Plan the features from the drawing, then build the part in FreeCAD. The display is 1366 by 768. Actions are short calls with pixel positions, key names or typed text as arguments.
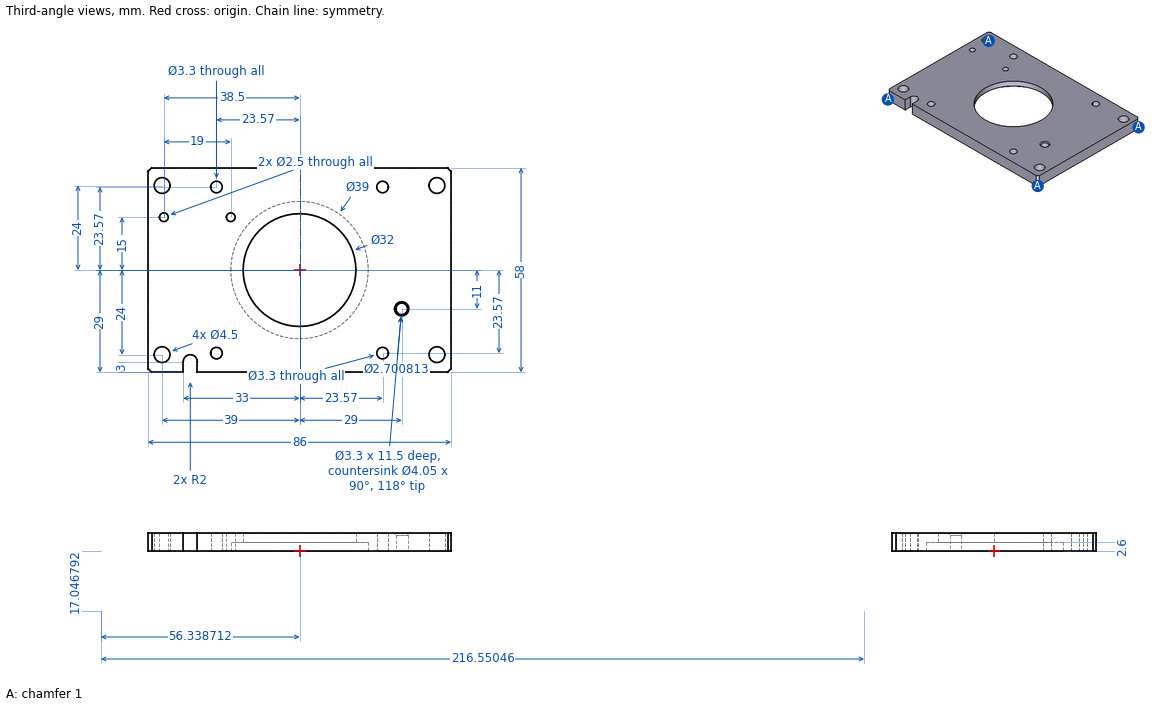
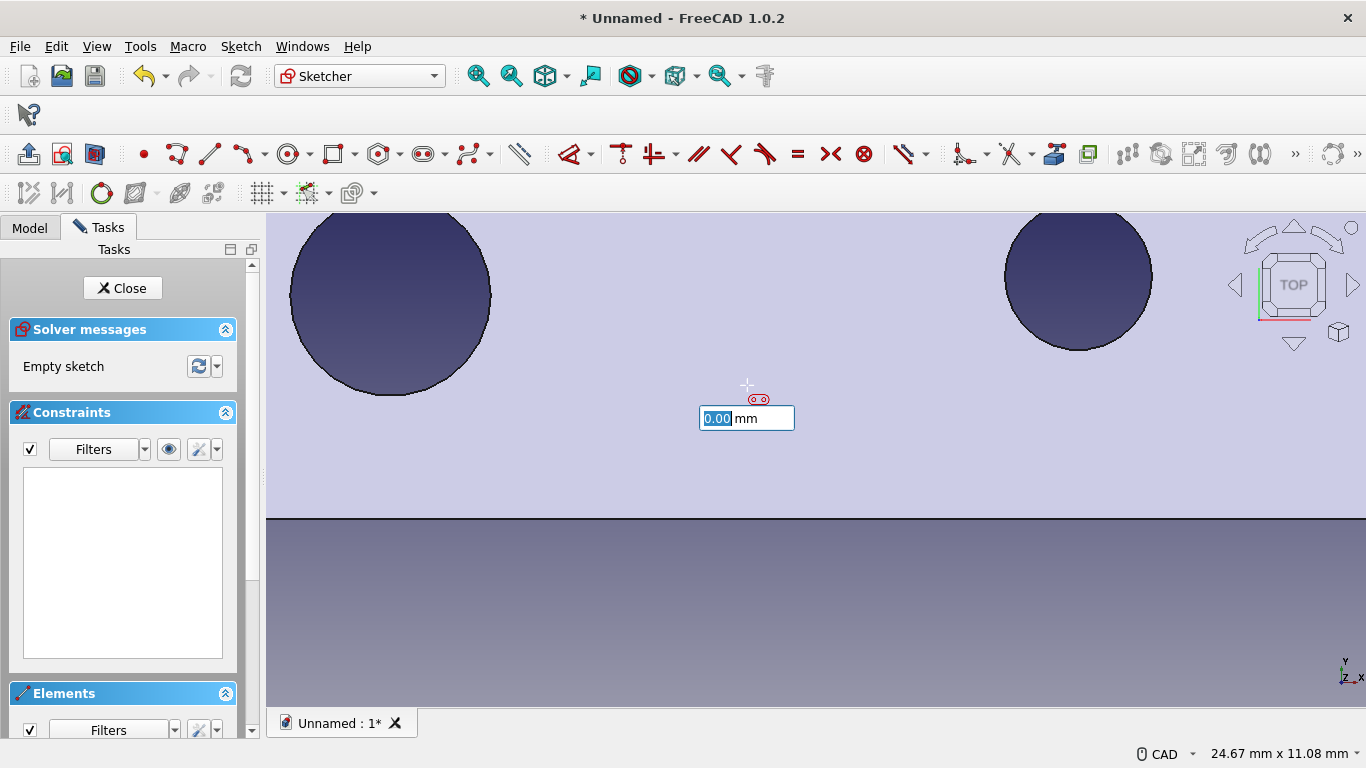
click(658, 452)
key(Escape)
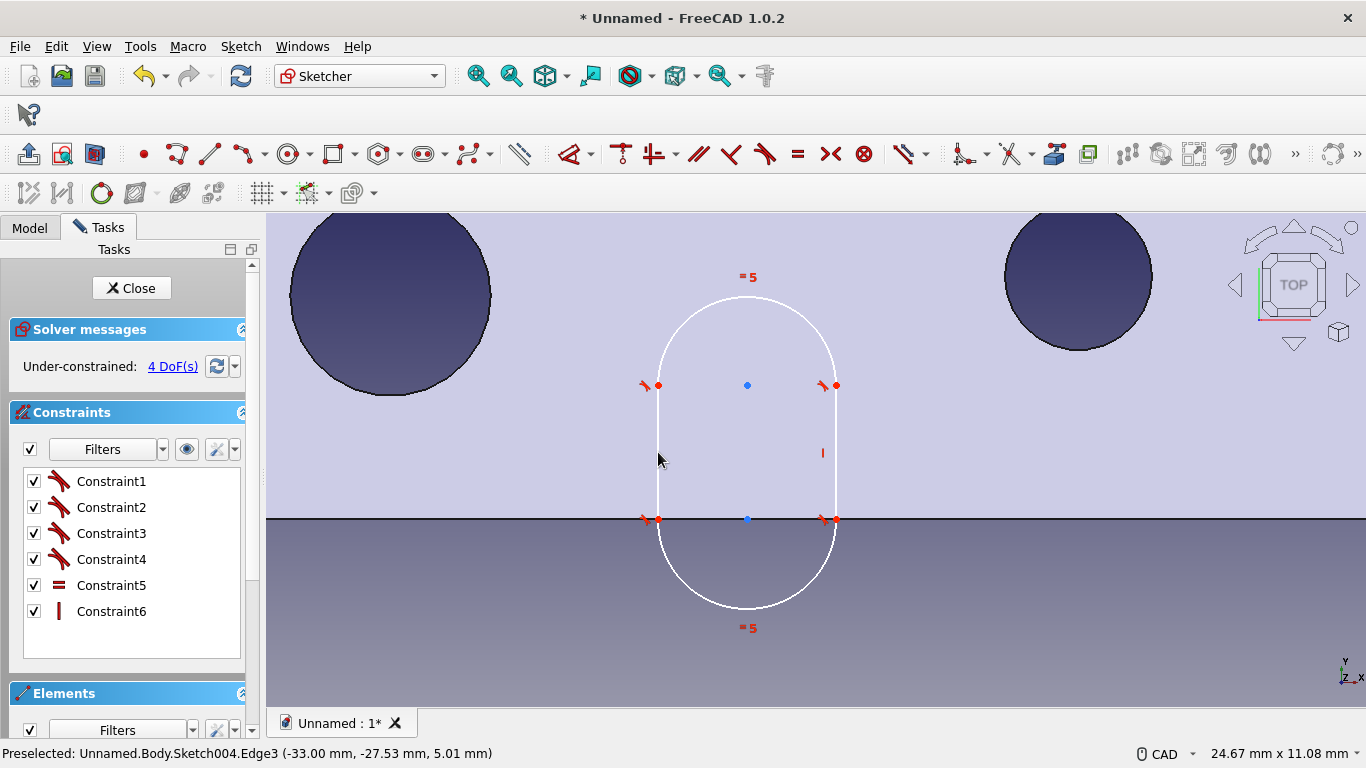
key(d)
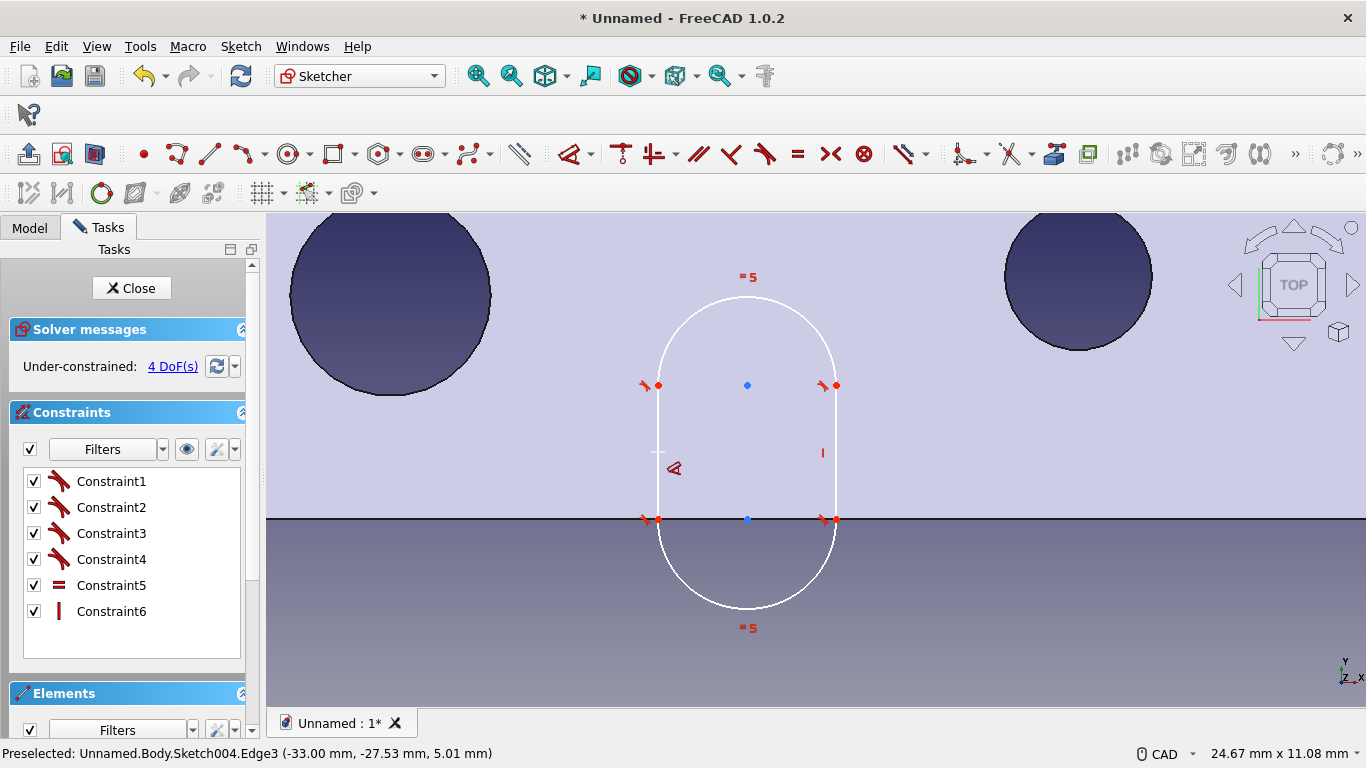
click(695, 592)
click(676, 618)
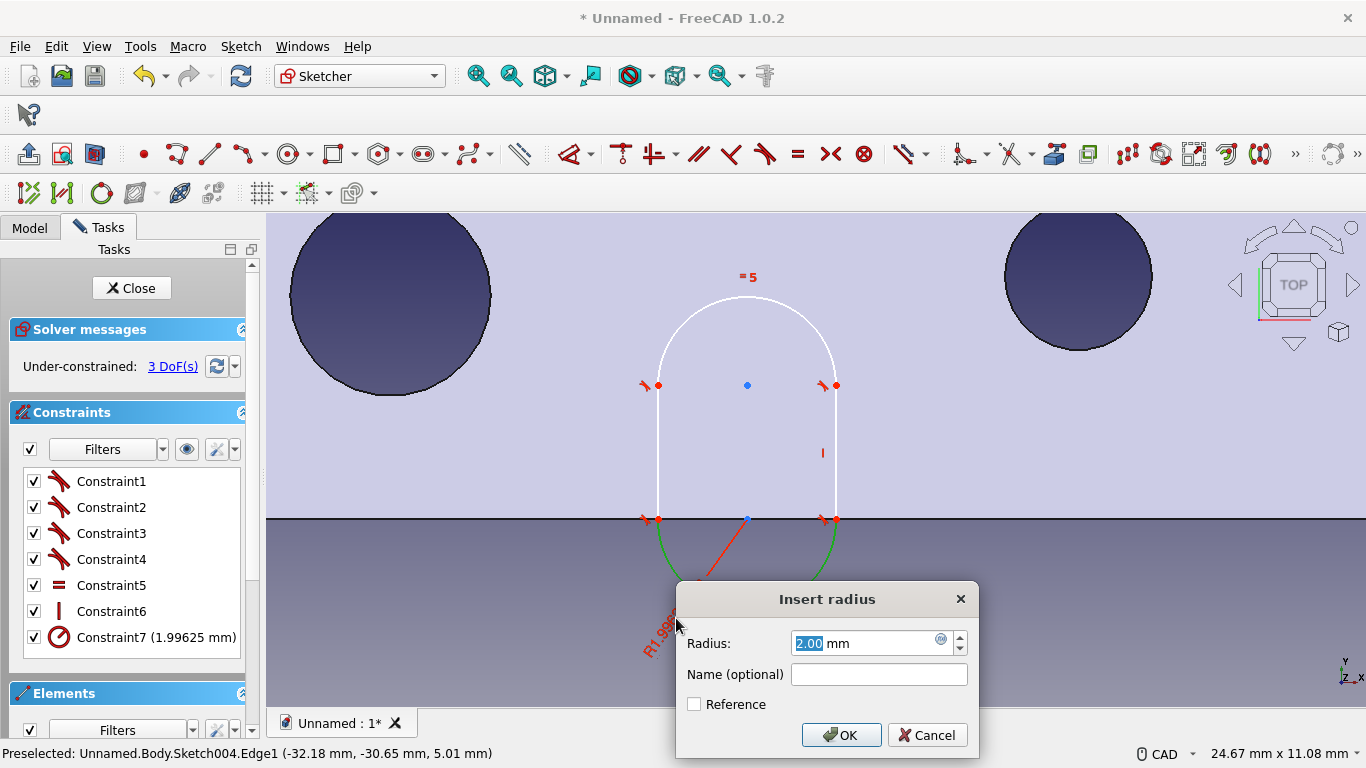
text(2)
key(Return)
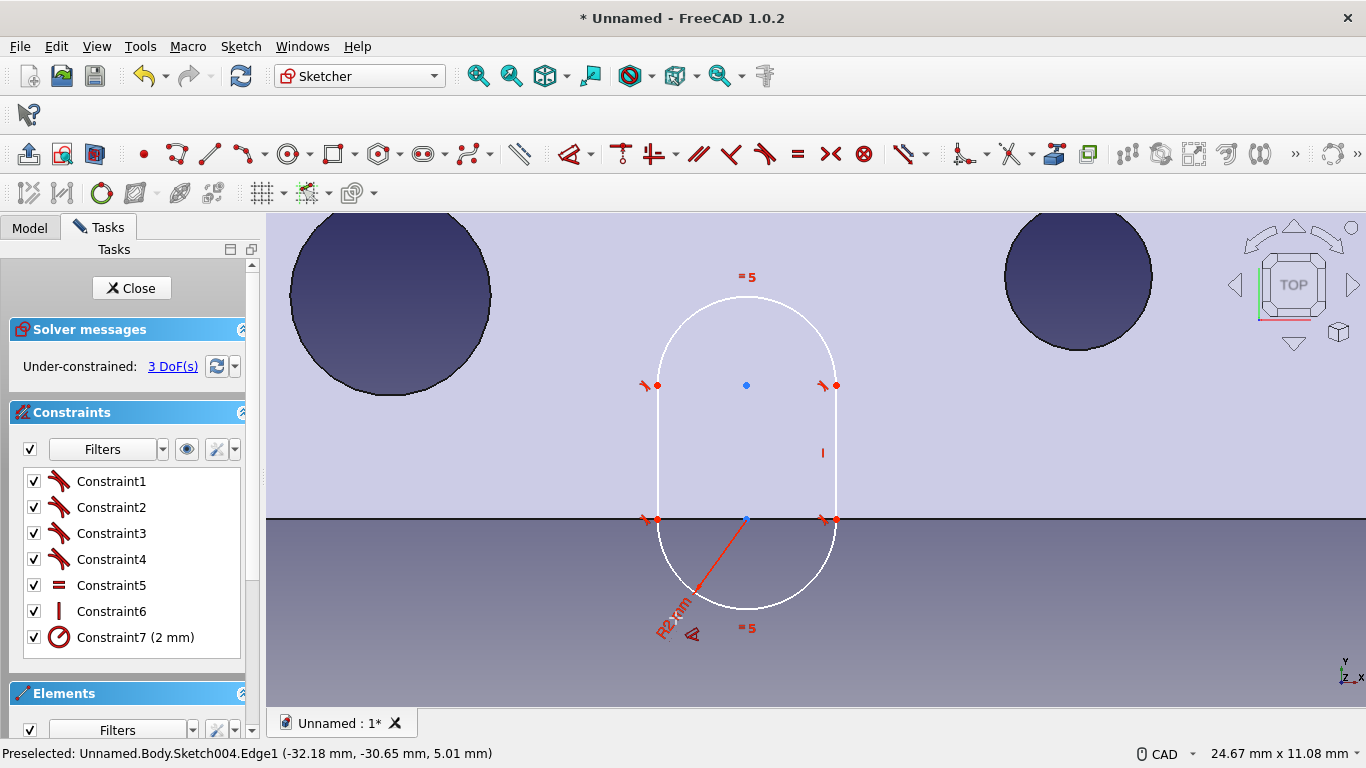
click(658, 480)
click(624, 453)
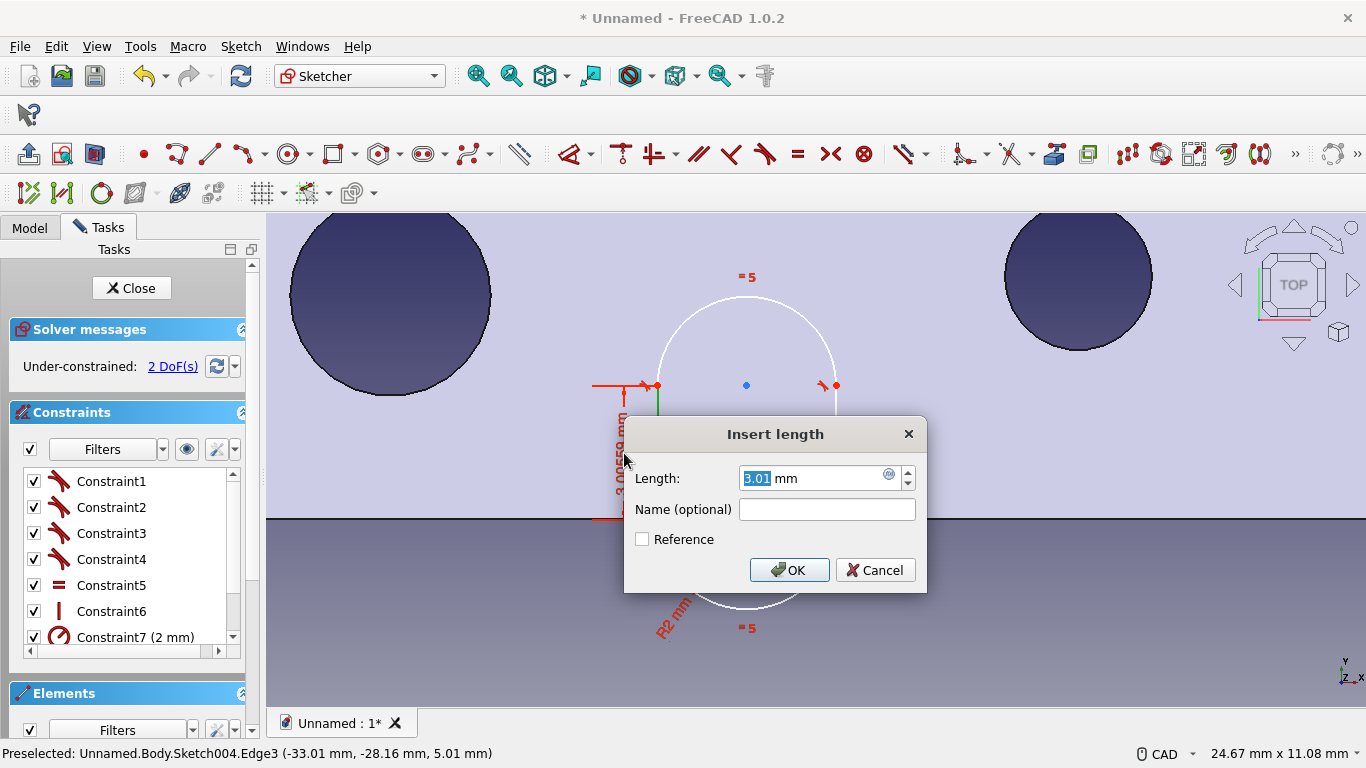
text(3)
key(Return)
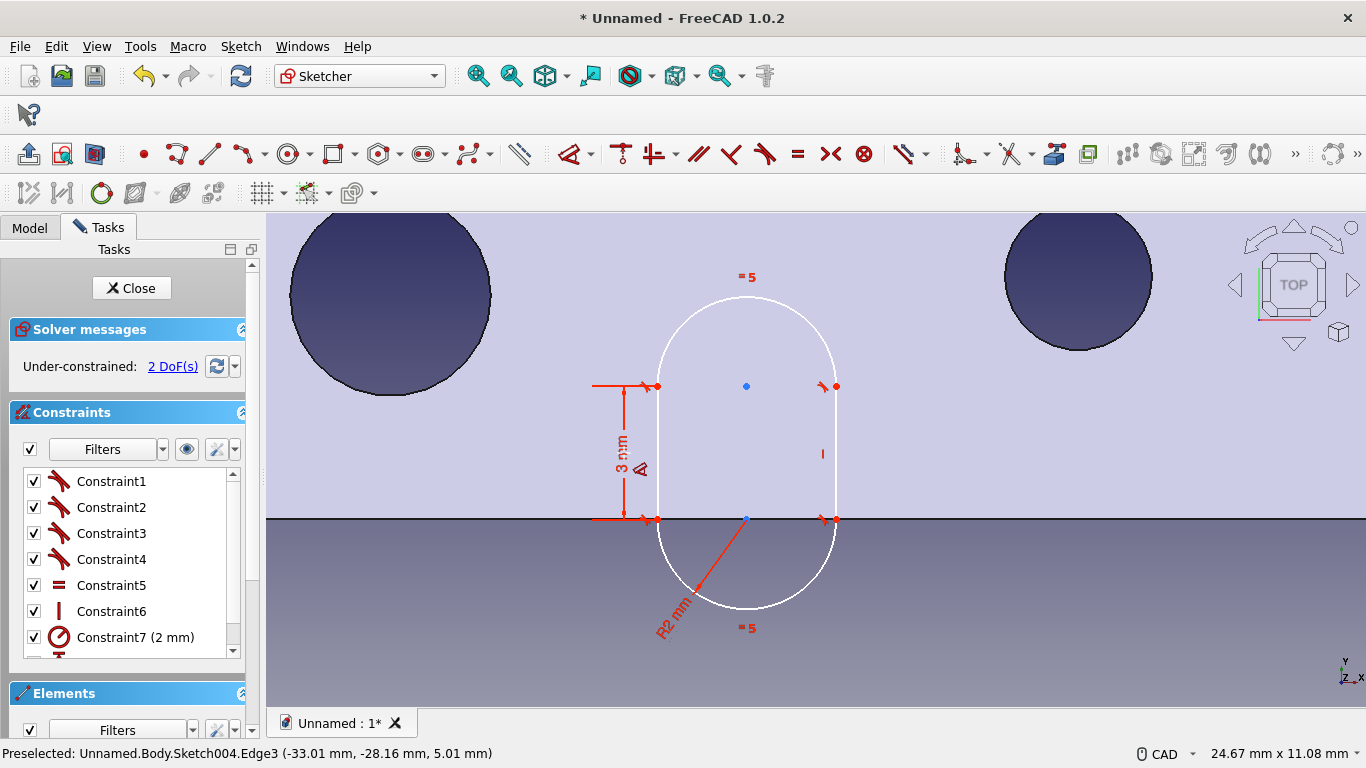
click(658, 520)
click(929, 554)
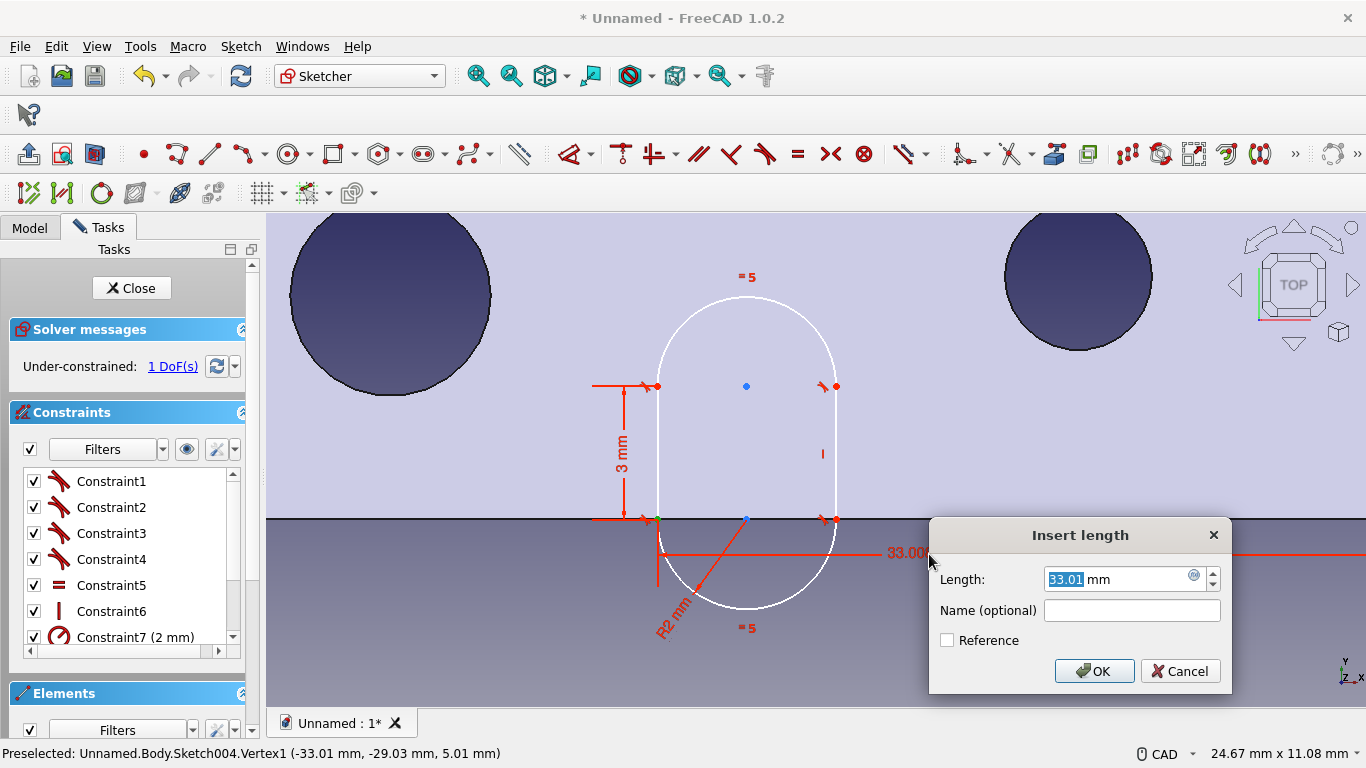
text(33)
key(Return)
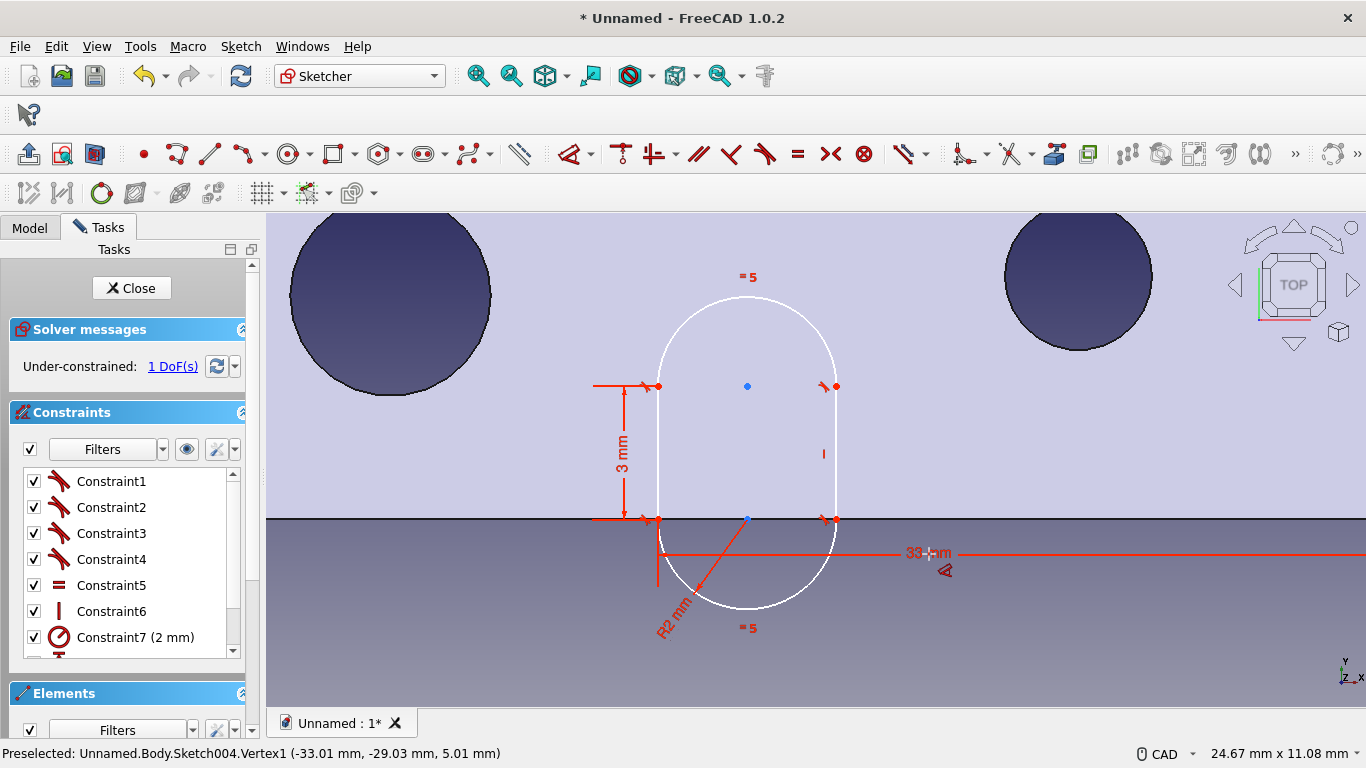
click(658, 520)
click(624, 380)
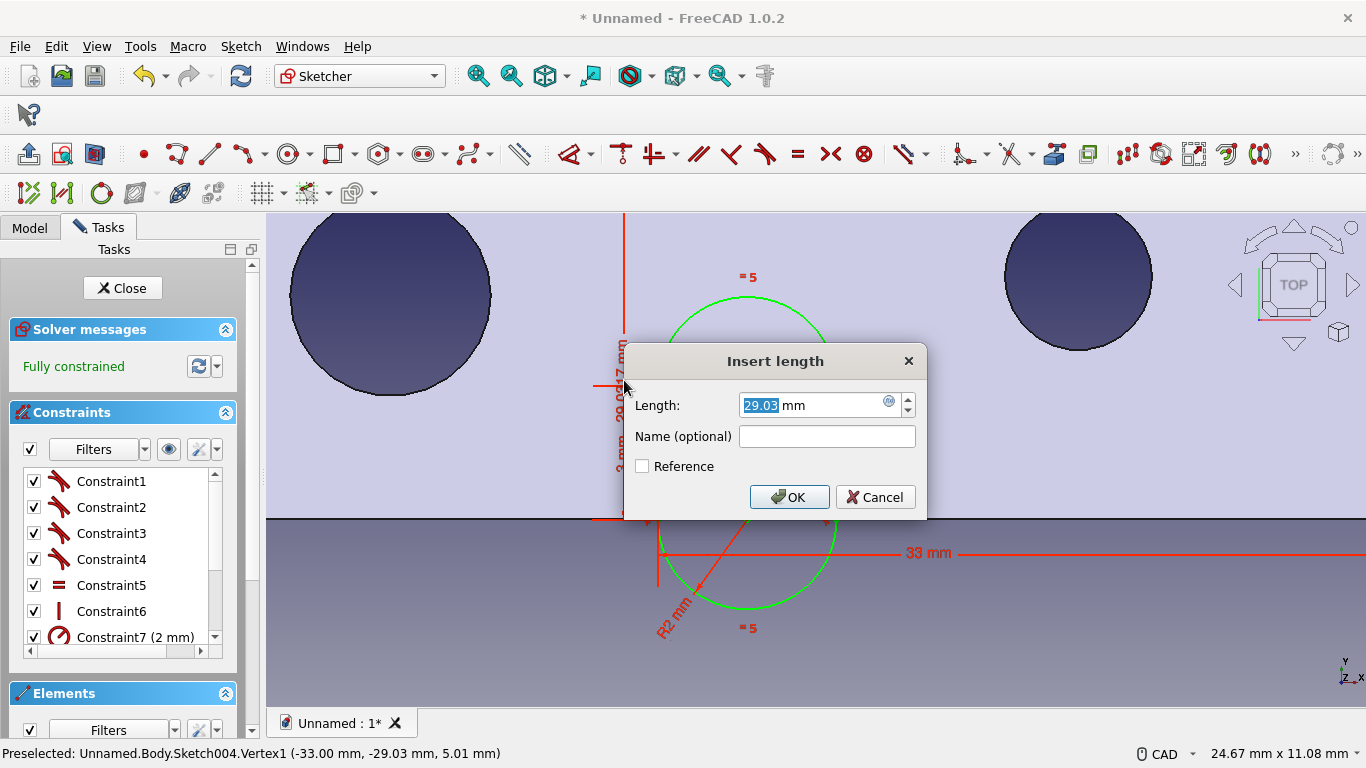
text(29)
key(Return)
key(Escape)